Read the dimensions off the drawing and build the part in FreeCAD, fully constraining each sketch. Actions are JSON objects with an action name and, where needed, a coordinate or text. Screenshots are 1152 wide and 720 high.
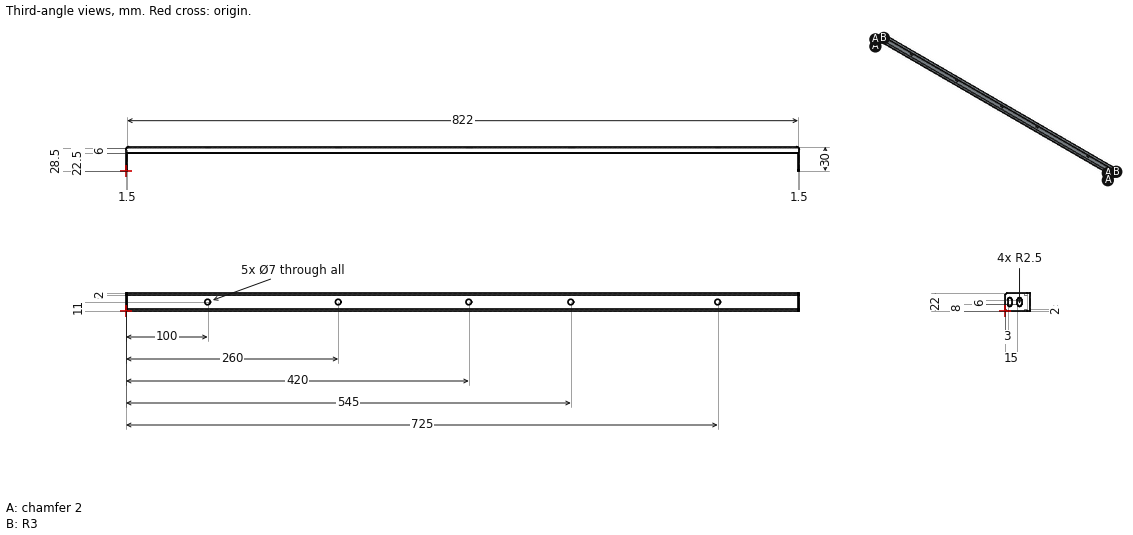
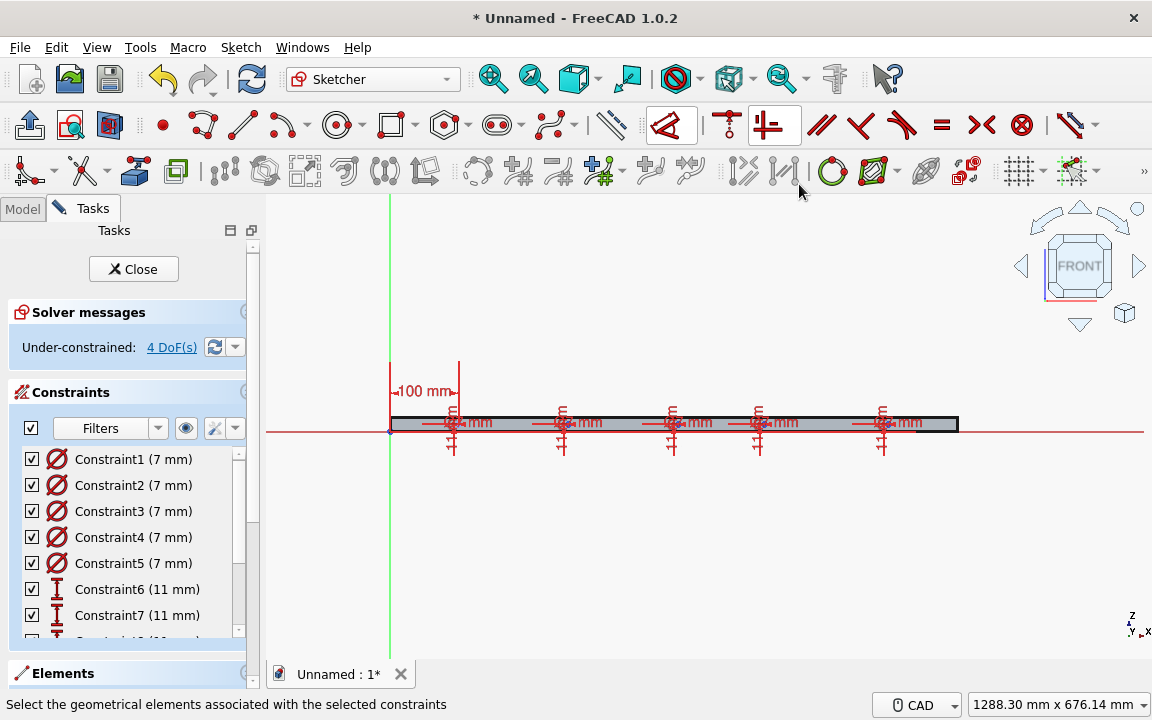
{"action": "left_click", "coordinate": [569, 424]}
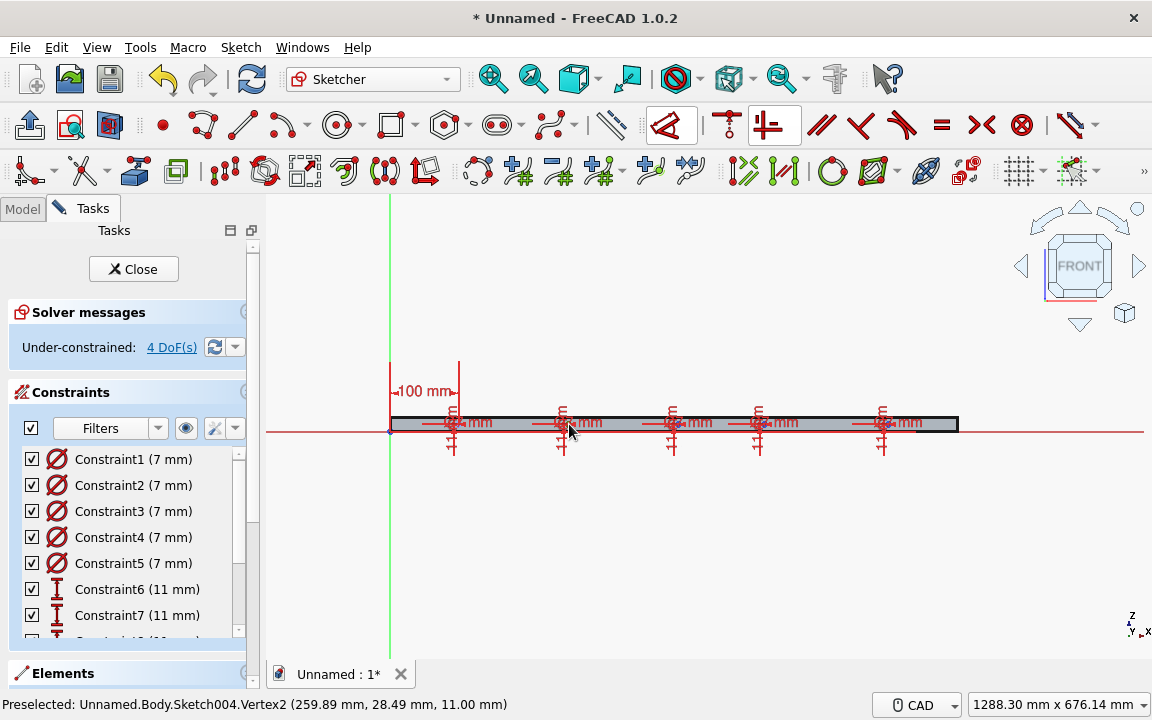
{"action": "left_click", "coordinate": [692, 126]}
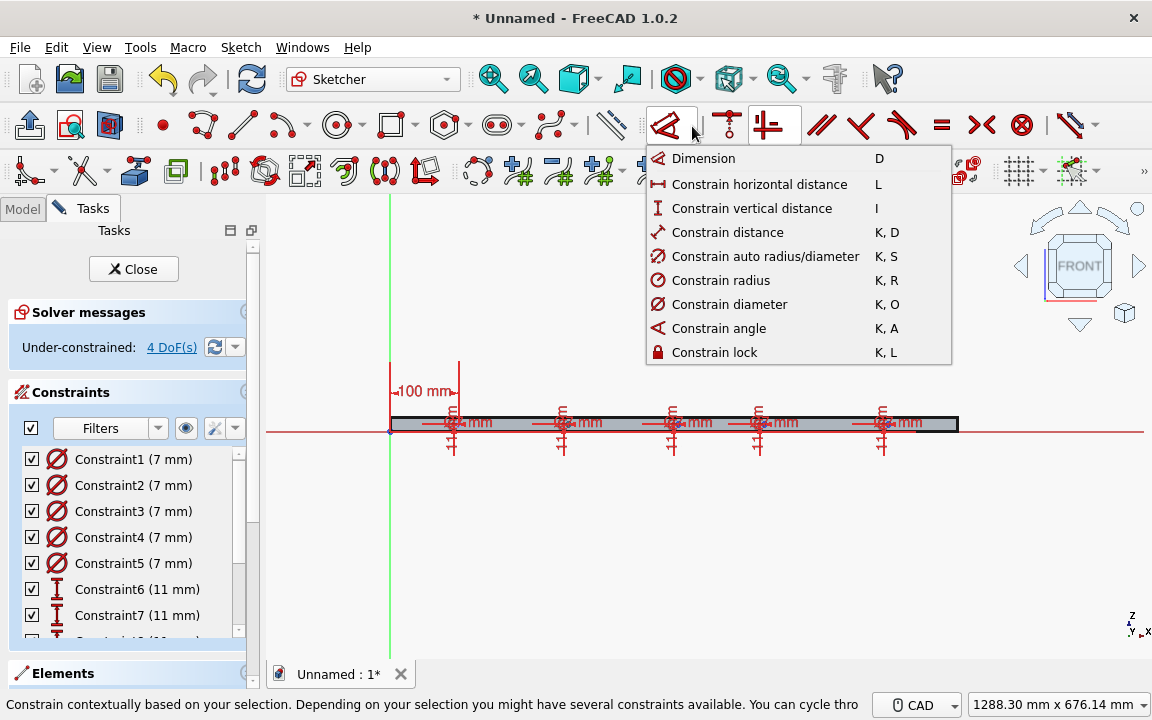
{"action": "left_click", "coordinate": [799, 184]}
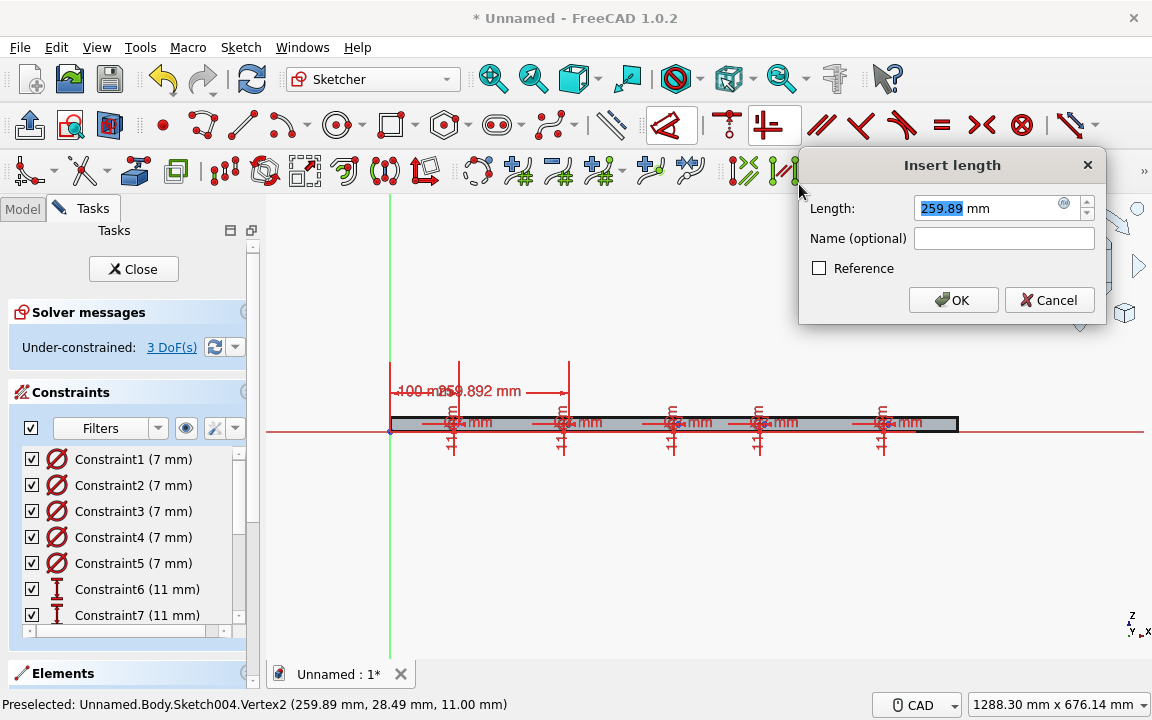
{"action": "type", "text": "260"}
{"action": "key", "text": "Return"}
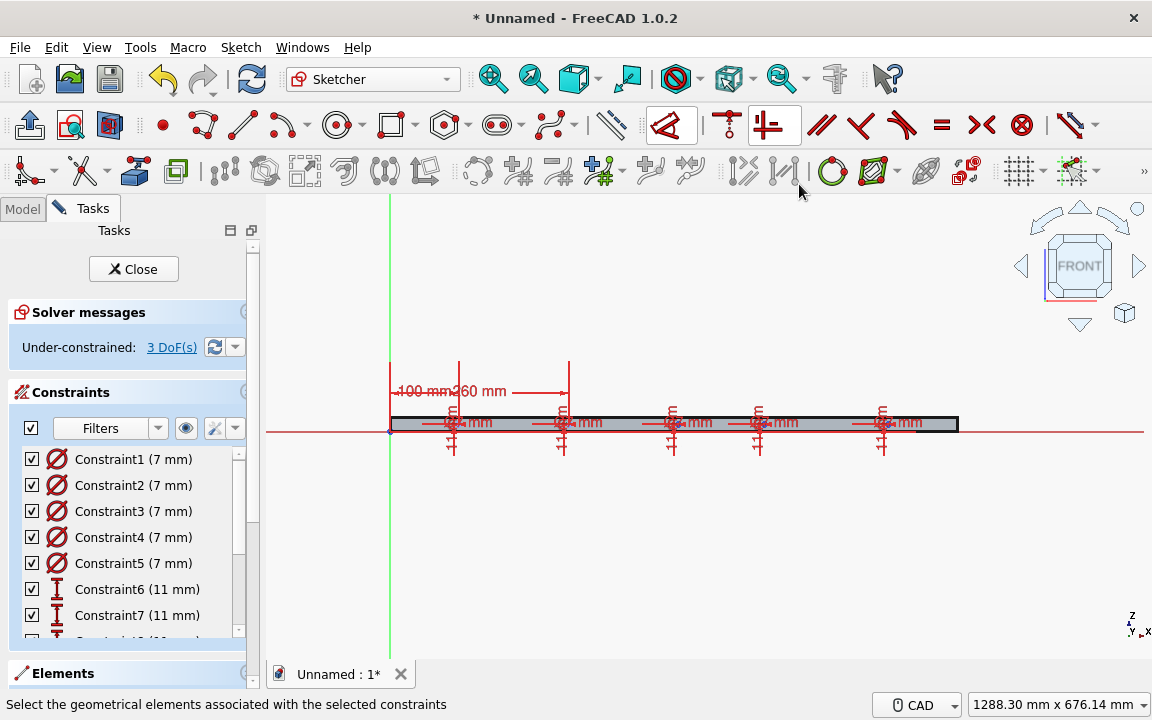
{"action": "left_click", "coordinate": [679, 424]}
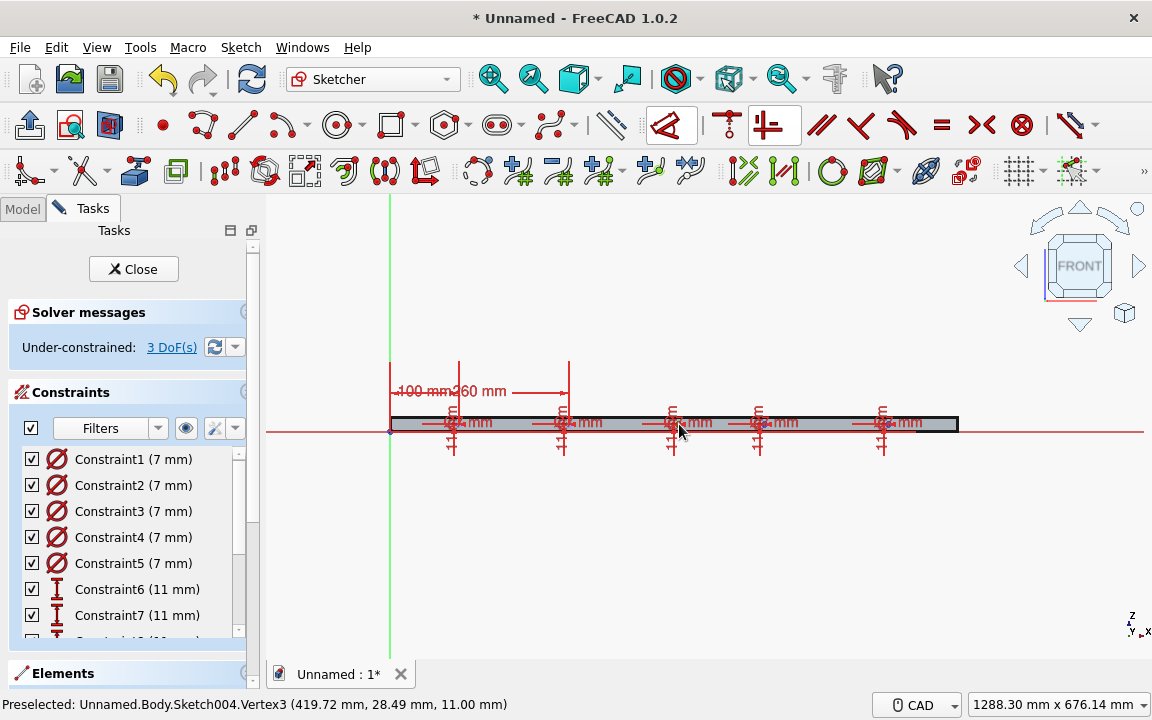
{"action": "key", "text": "l"}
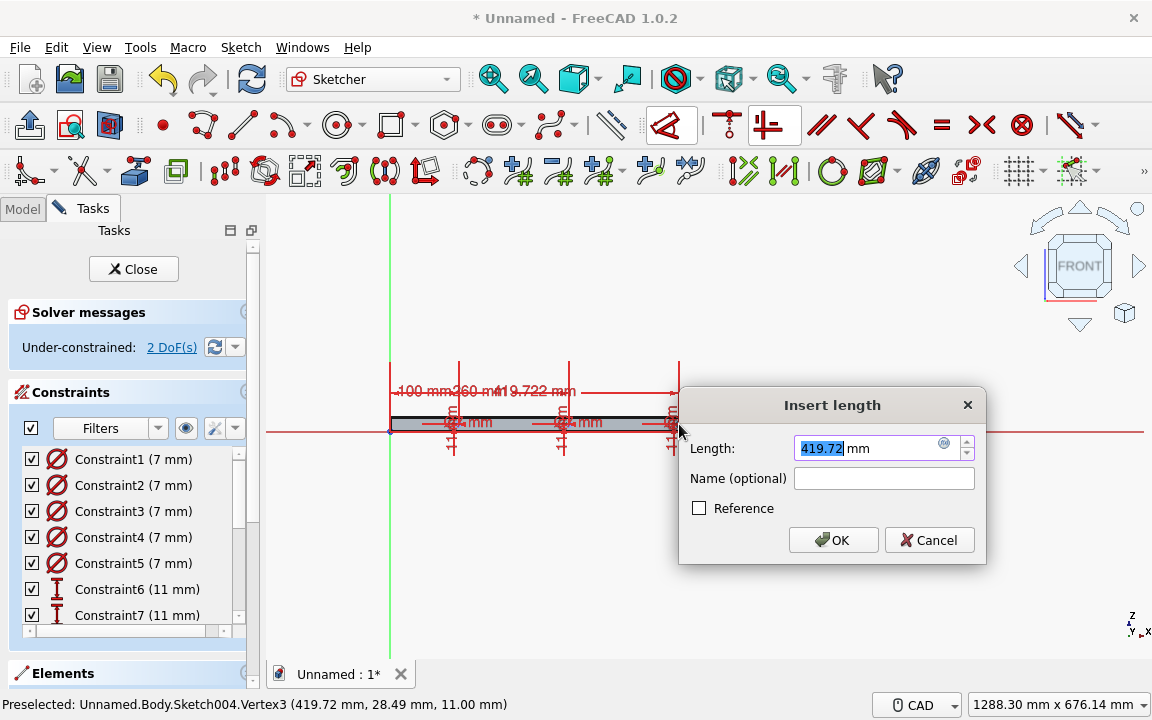
{"action": "type", "text": "420"}
{"action": "key", "text": "Return"}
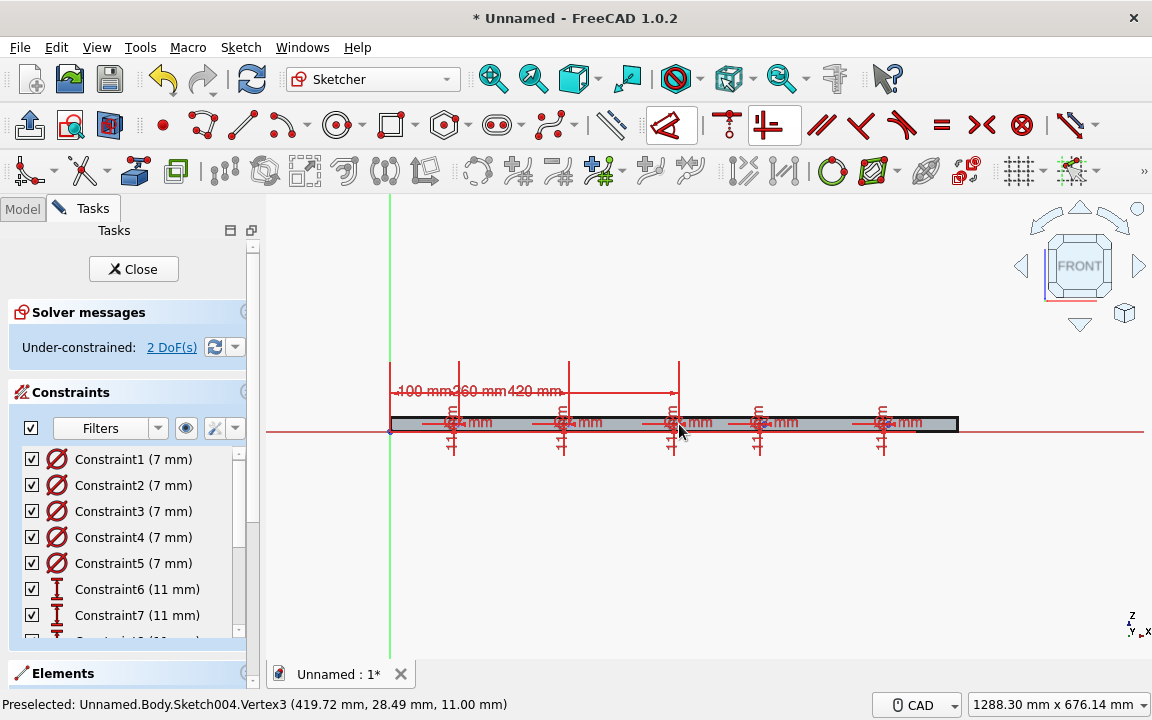
{"action": "left_click", "coordinate": [765, 424]}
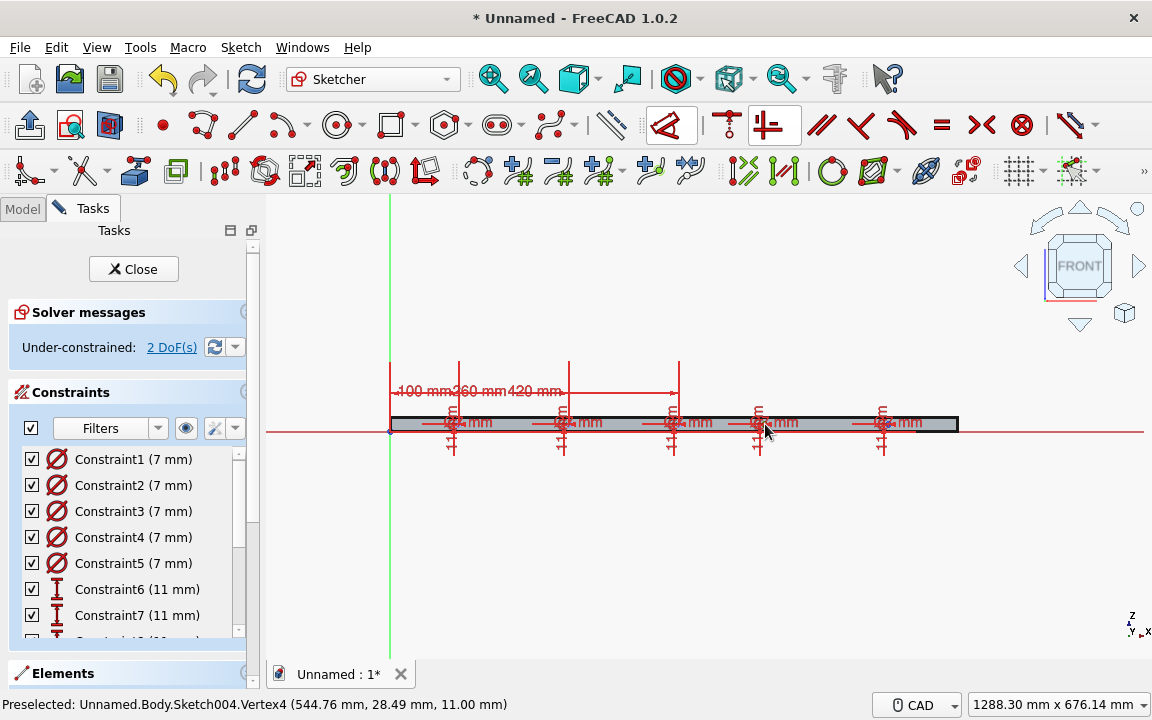
{"action": "key", "text": "l"}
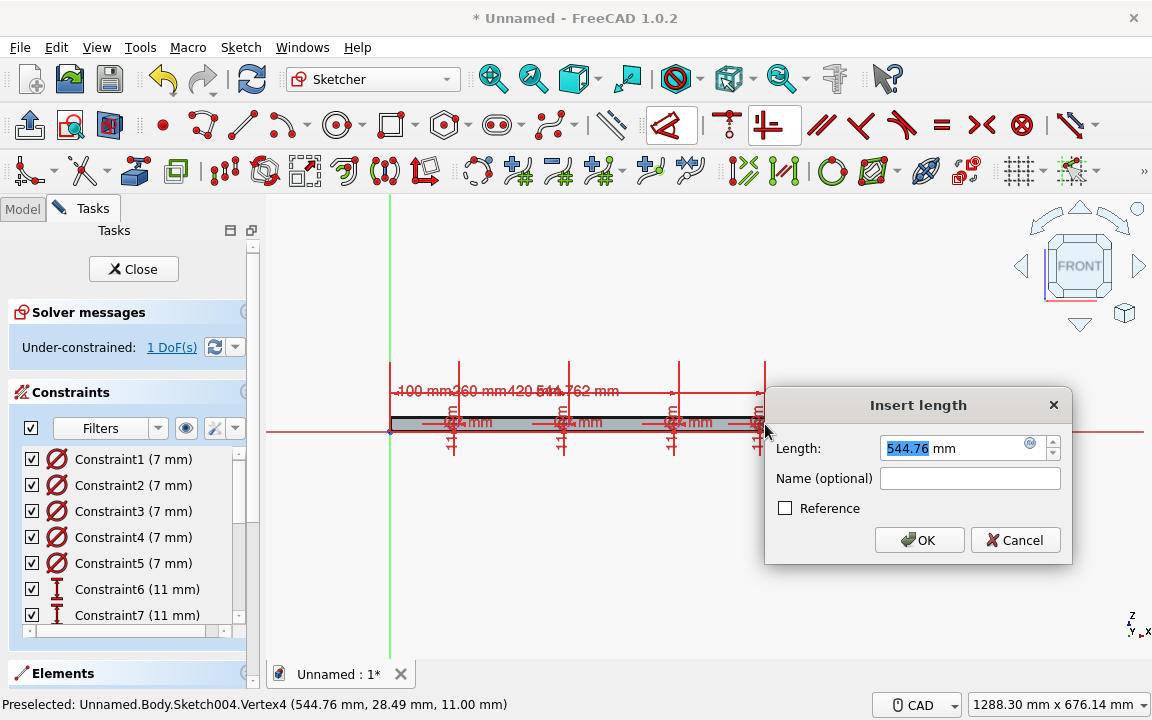
{"action": "type", "text": "545"}
{"action": "key", "text": "Return"}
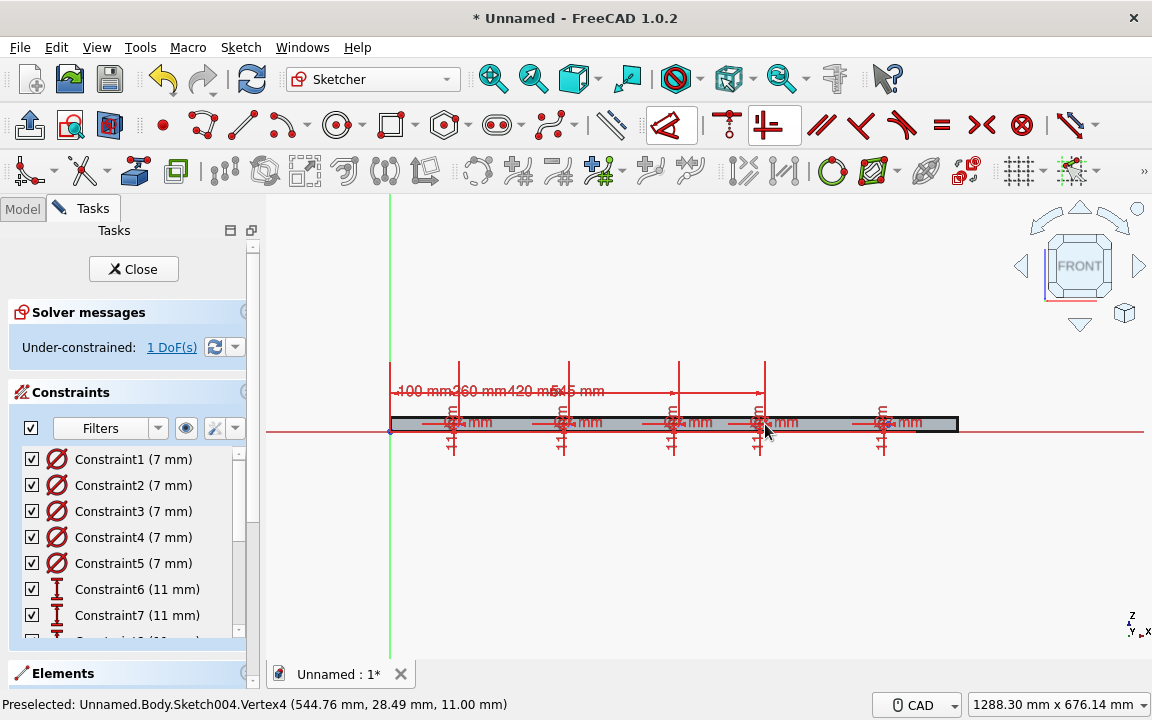
{"action": "left_click", "coordinate": [889, 424]}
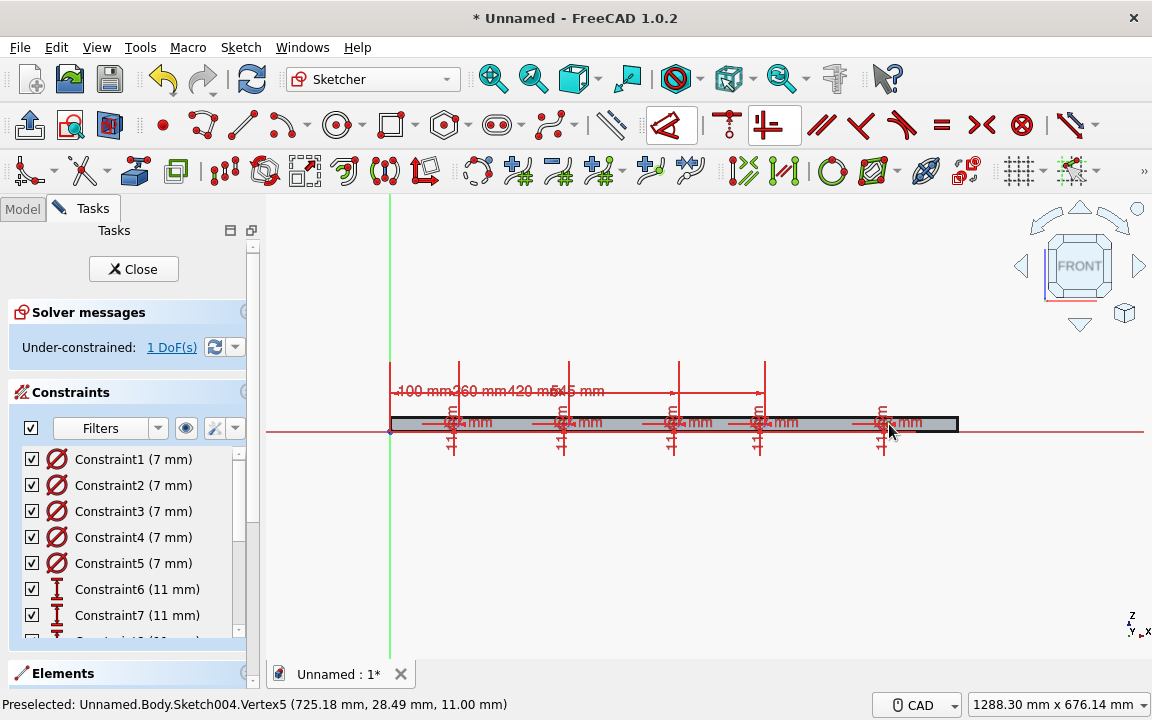
{"action": "key", "text": "l"}